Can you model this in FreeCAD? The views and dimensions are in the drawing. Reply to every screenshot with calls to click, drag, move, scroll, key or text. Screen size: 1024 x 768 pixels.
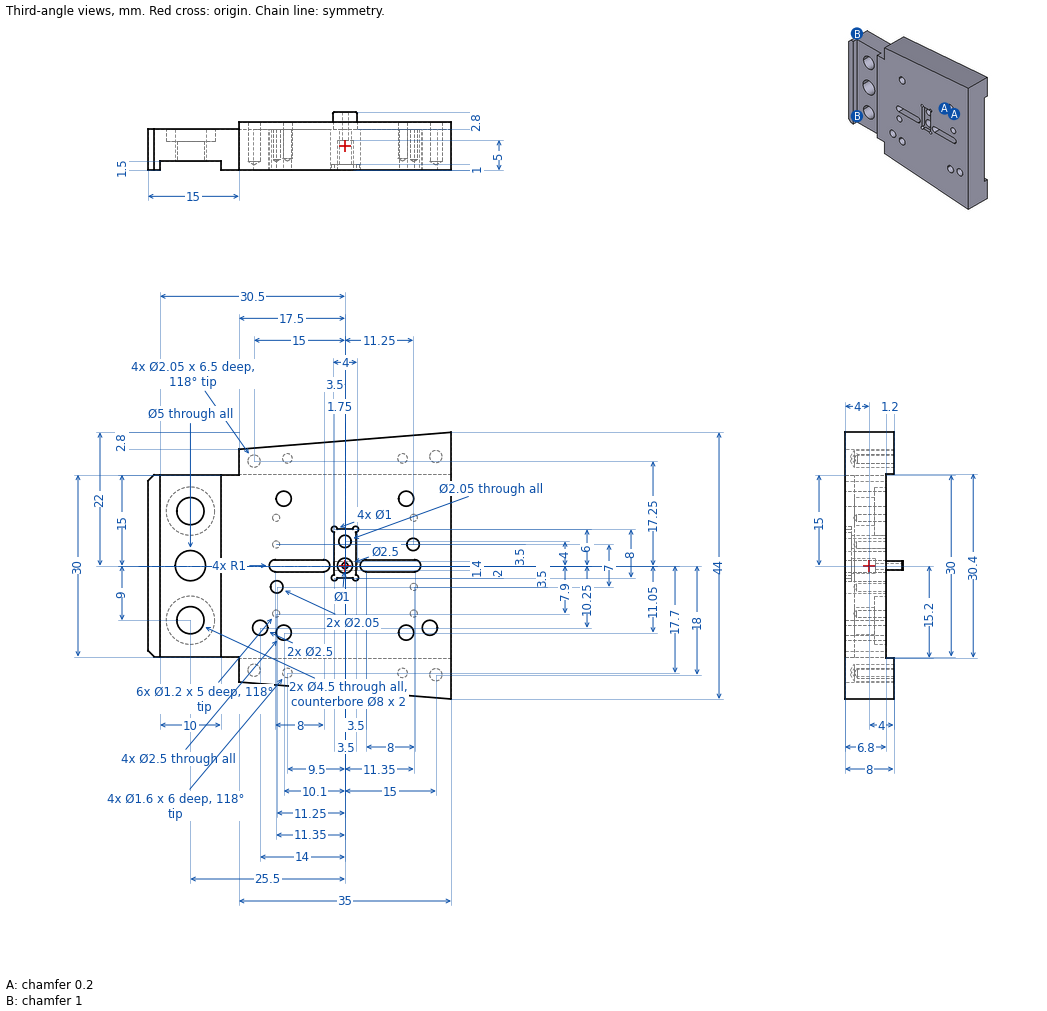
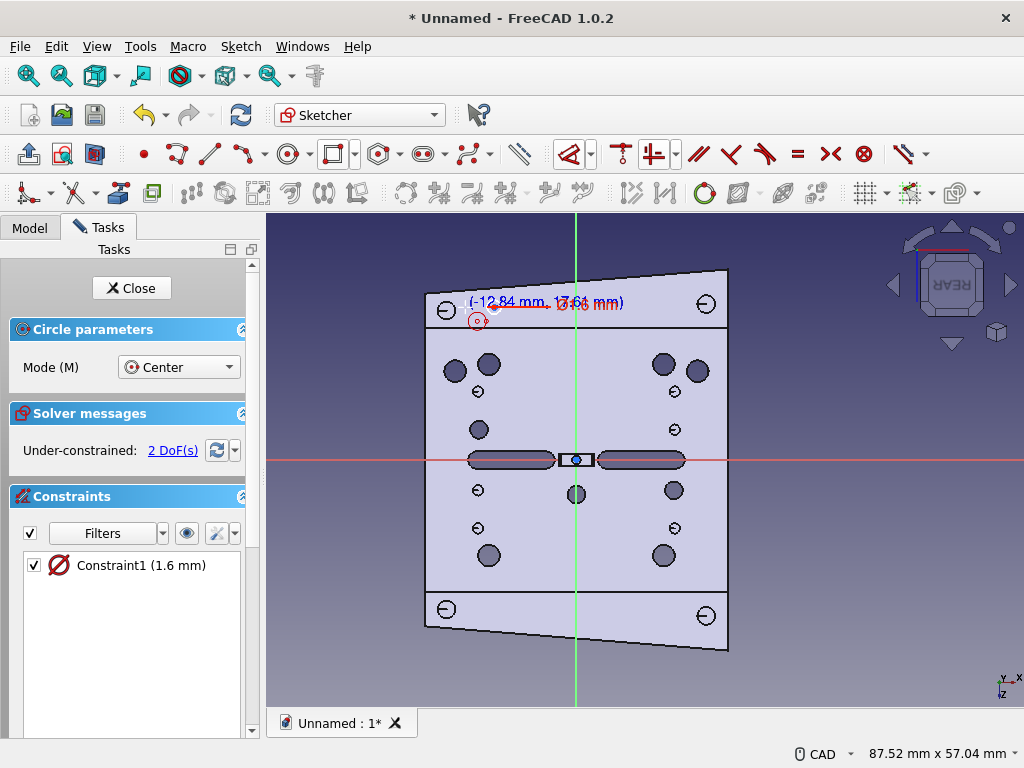
scroll(659, 307, up, 6)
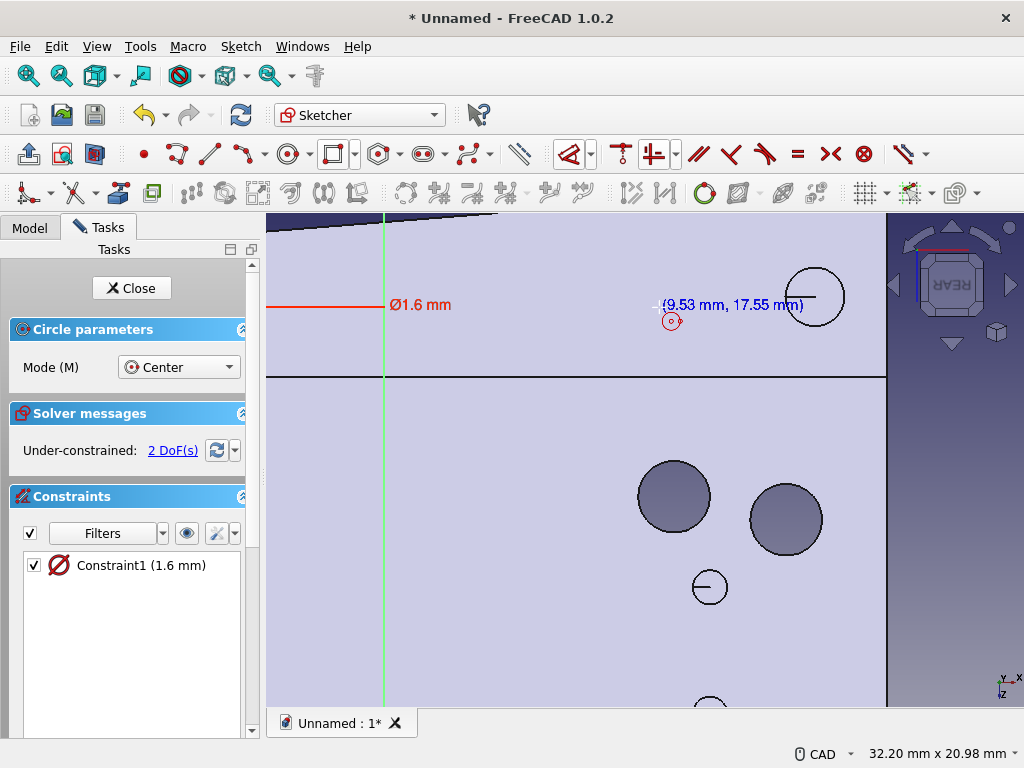
click(657, 306)
move(673, 289)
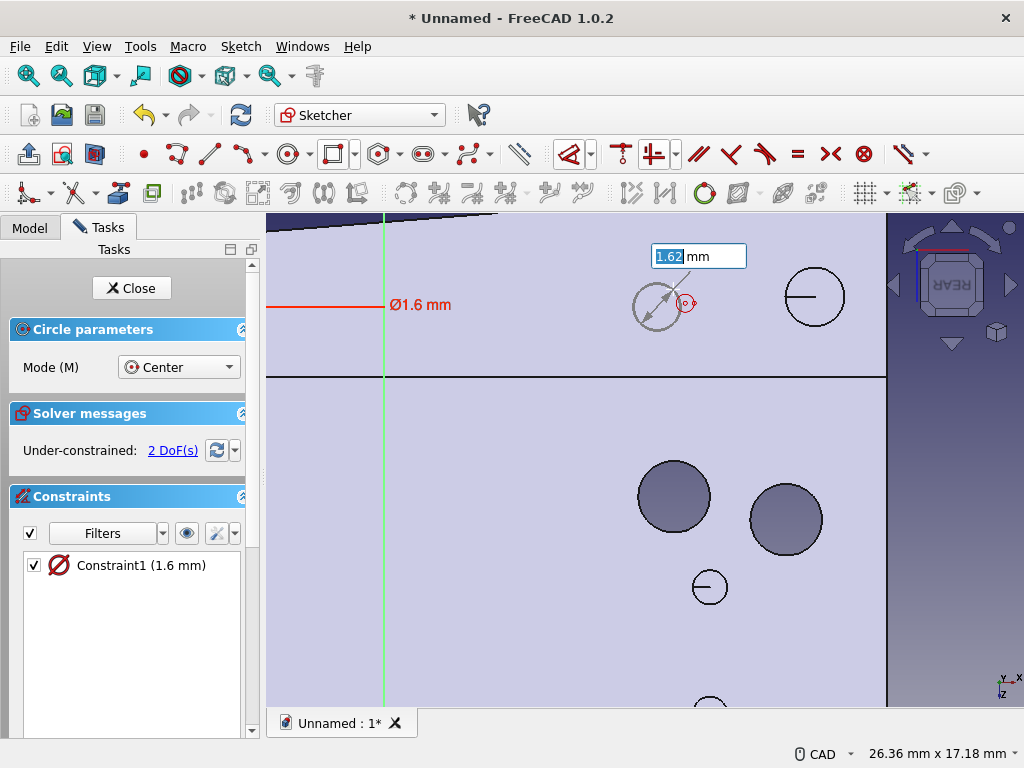
text(1.6)
key(Return)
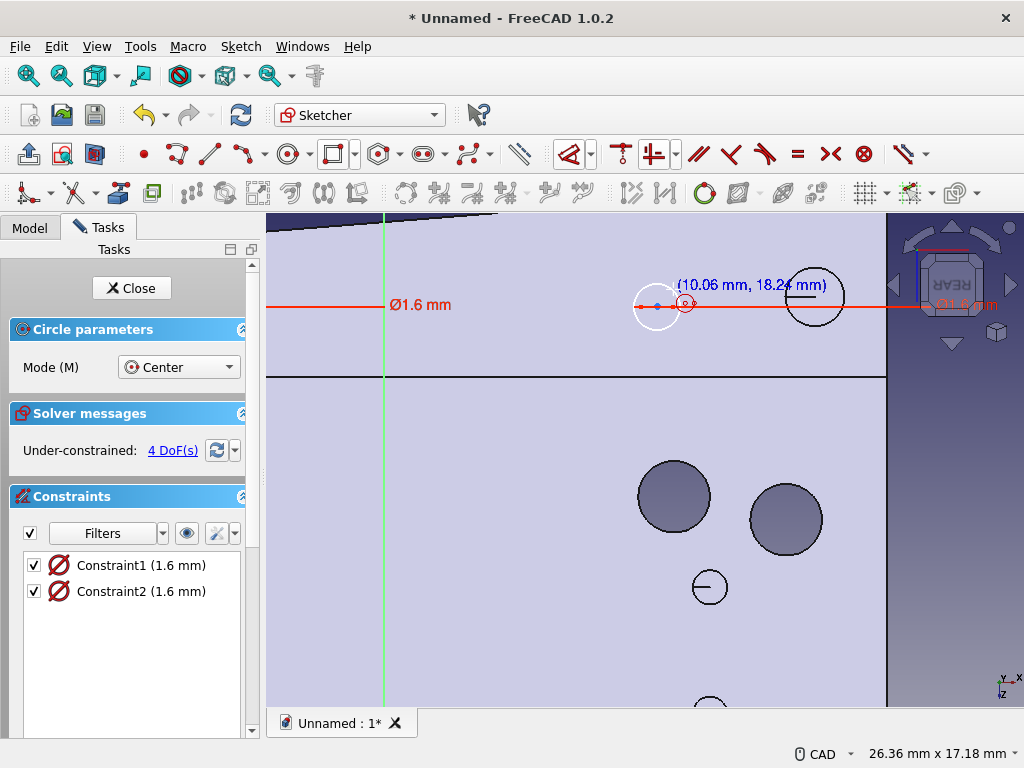
scroll(660, 307, down, 6)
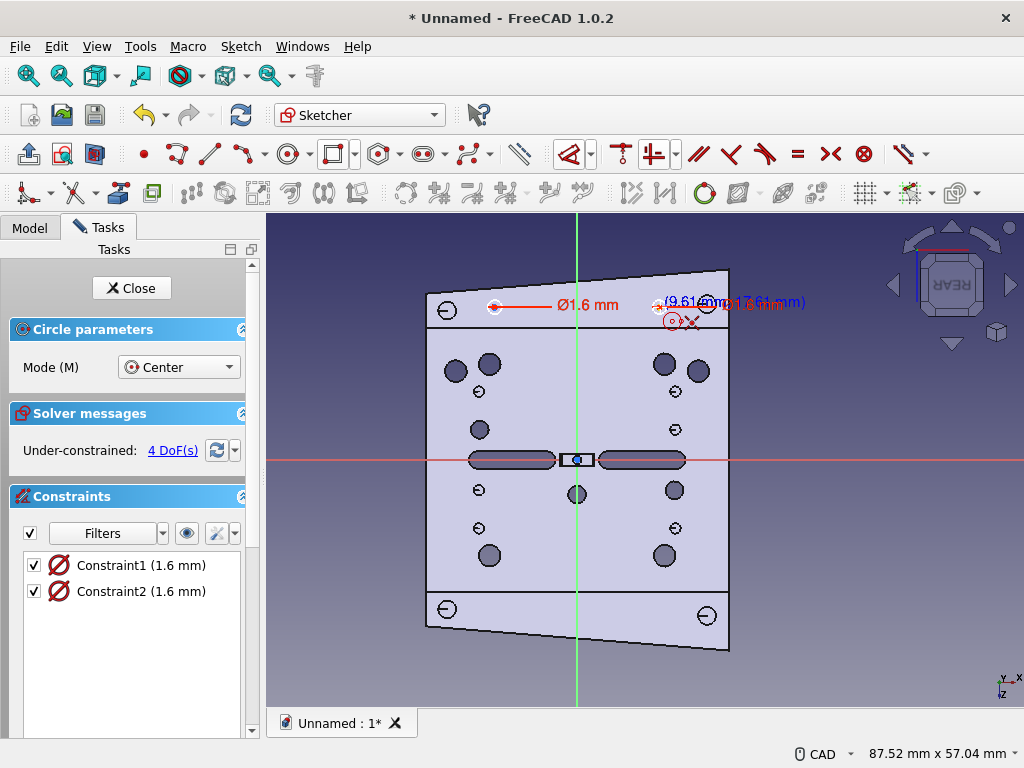
scroll(659, 613, up, 6)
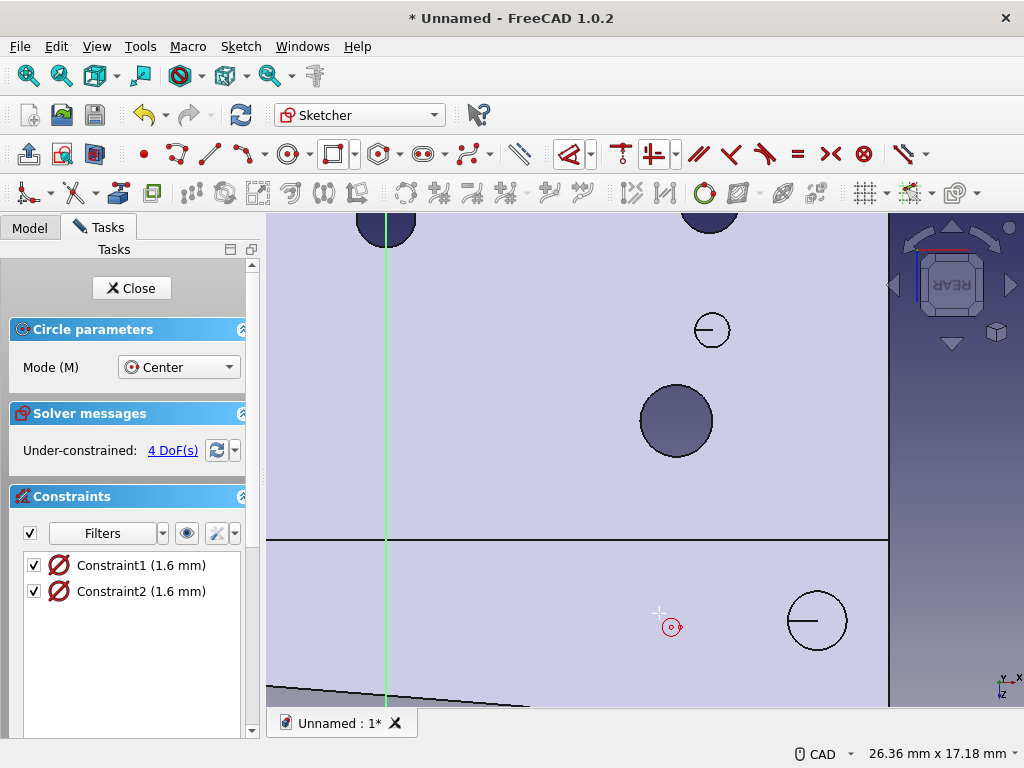
click(659, 612)
move(675, 596)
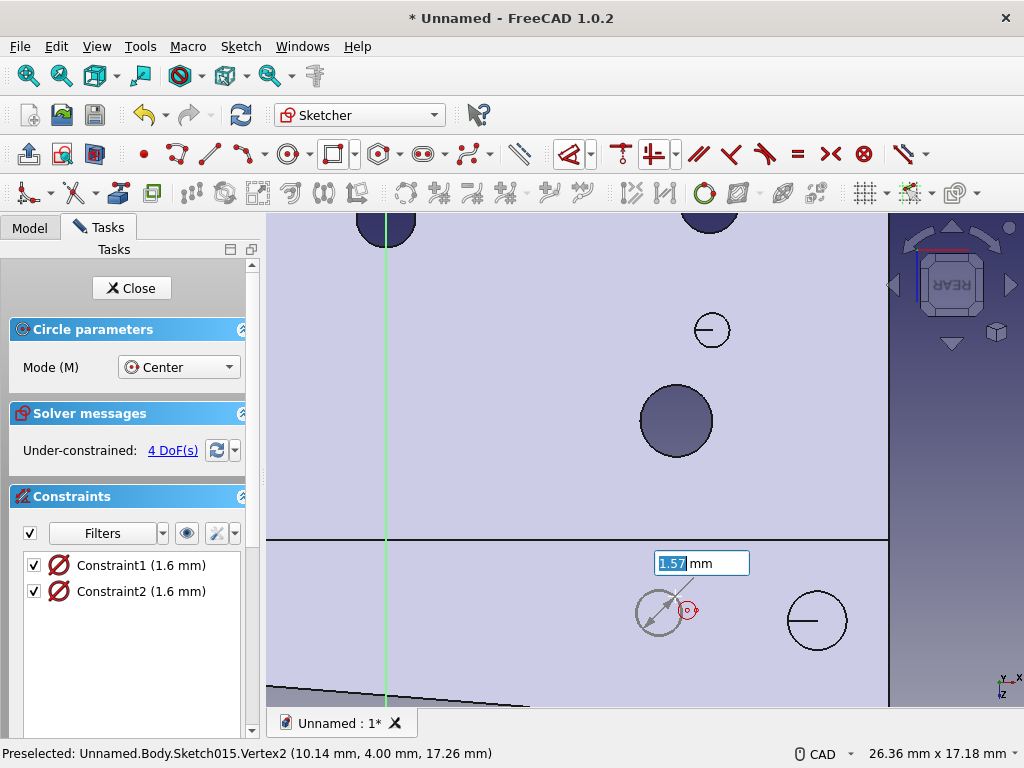
text(1.6)
key(Return)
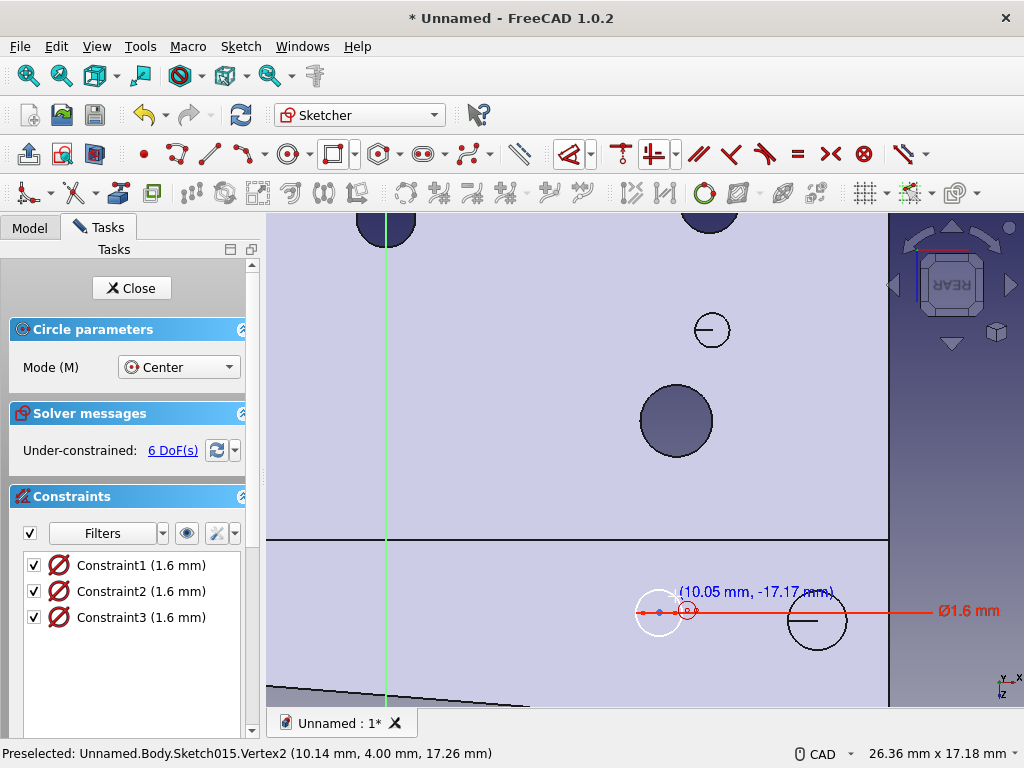
scroll(659, 614, down, 6)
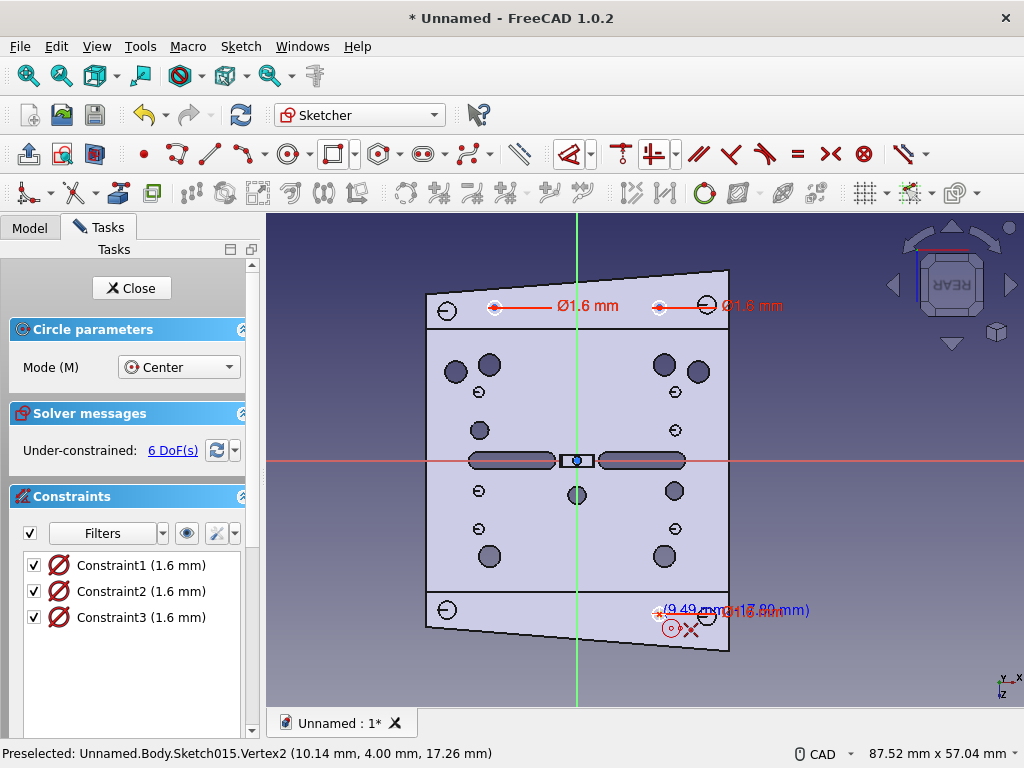
scroll(495, 614, up, 6)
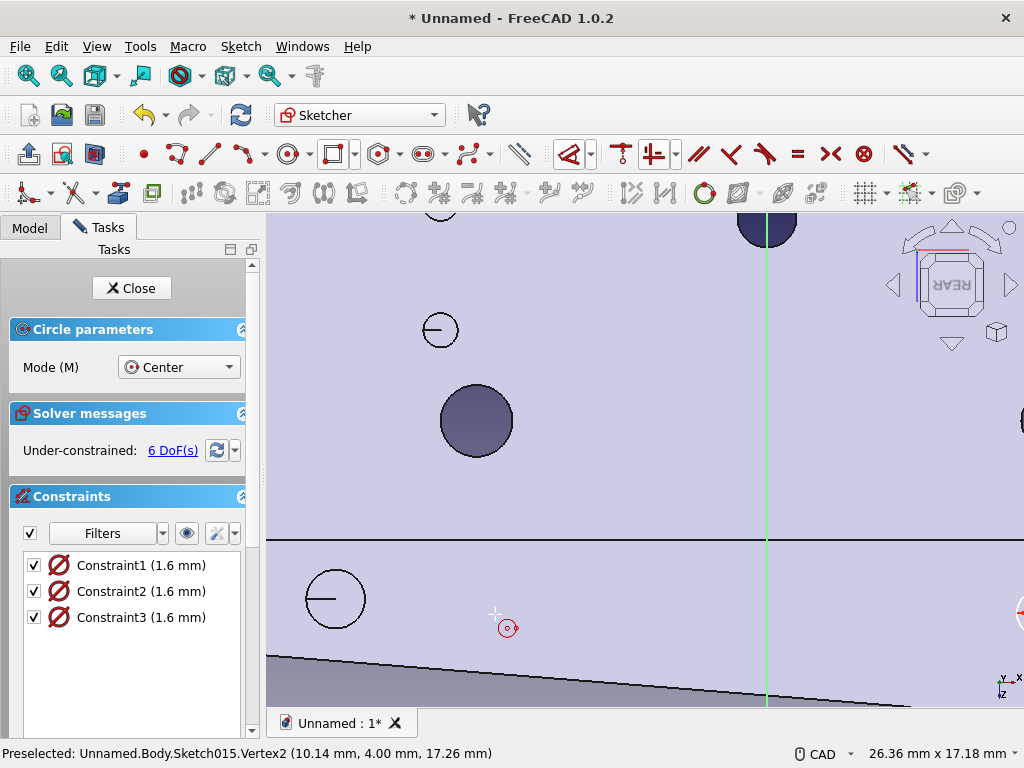
click(494, 612)
move(510, 596)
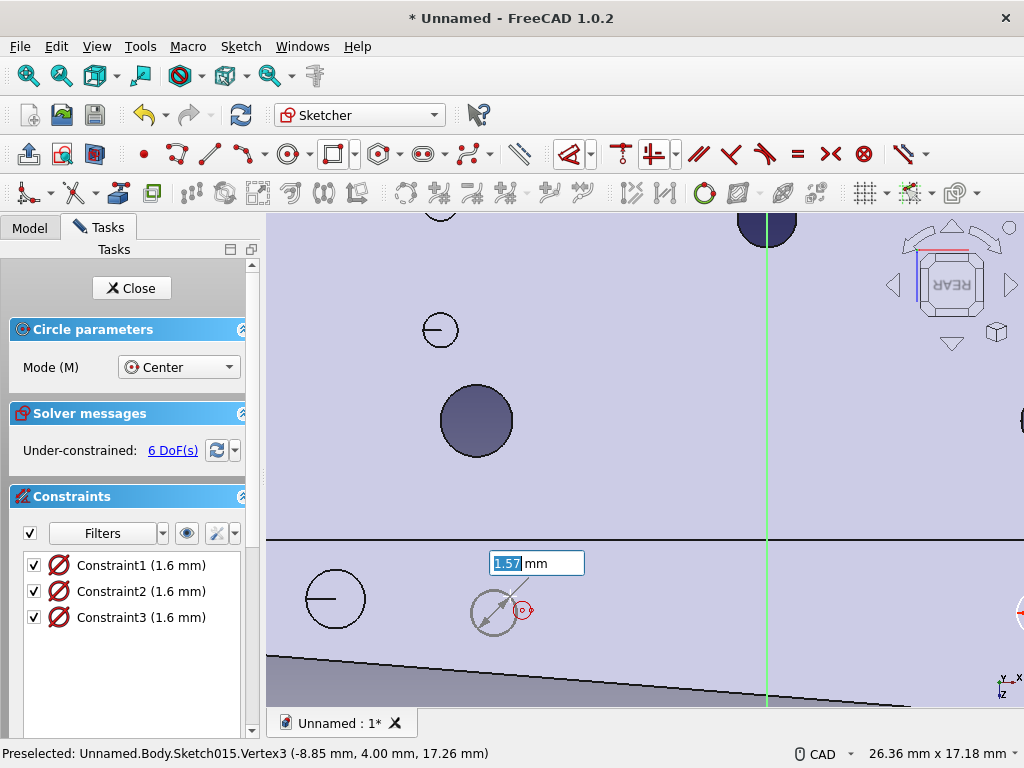
text(1.6)
key(Return)
key(Escape)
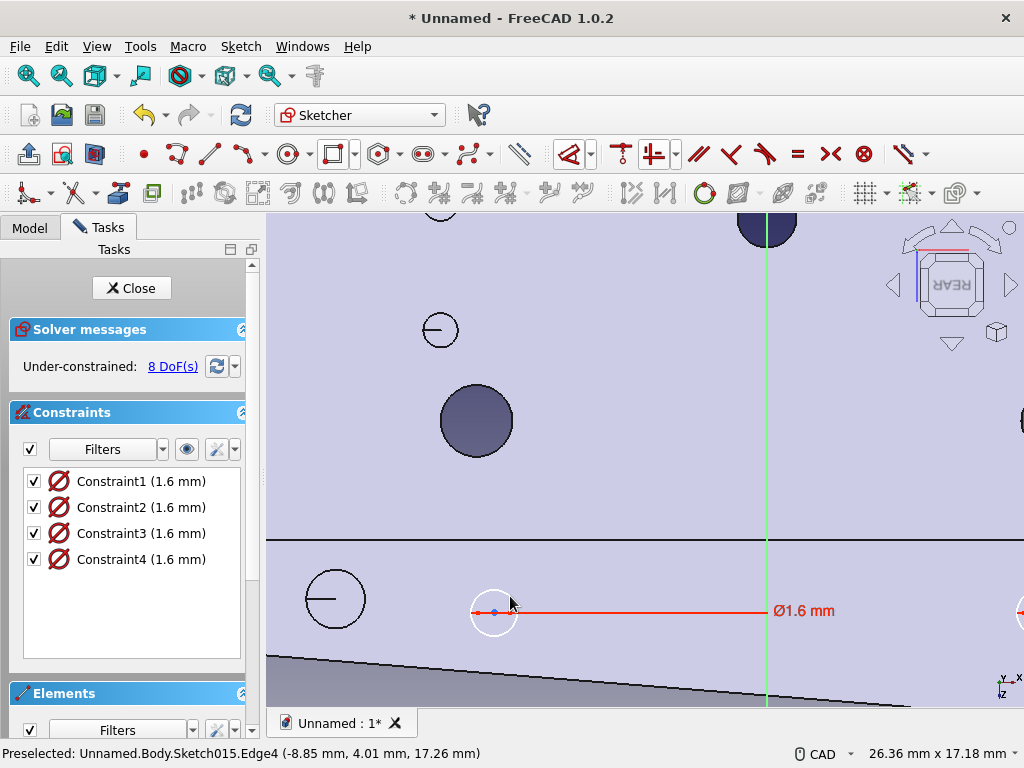
scroll(494, 614, down, 6)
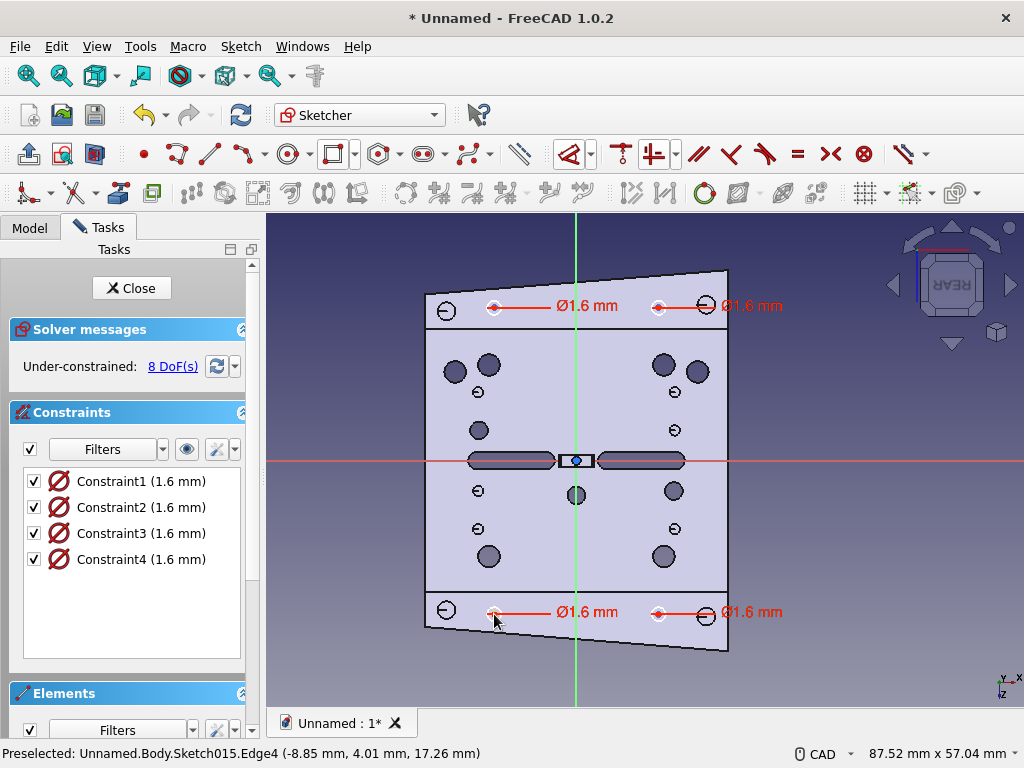
click(494, 308)